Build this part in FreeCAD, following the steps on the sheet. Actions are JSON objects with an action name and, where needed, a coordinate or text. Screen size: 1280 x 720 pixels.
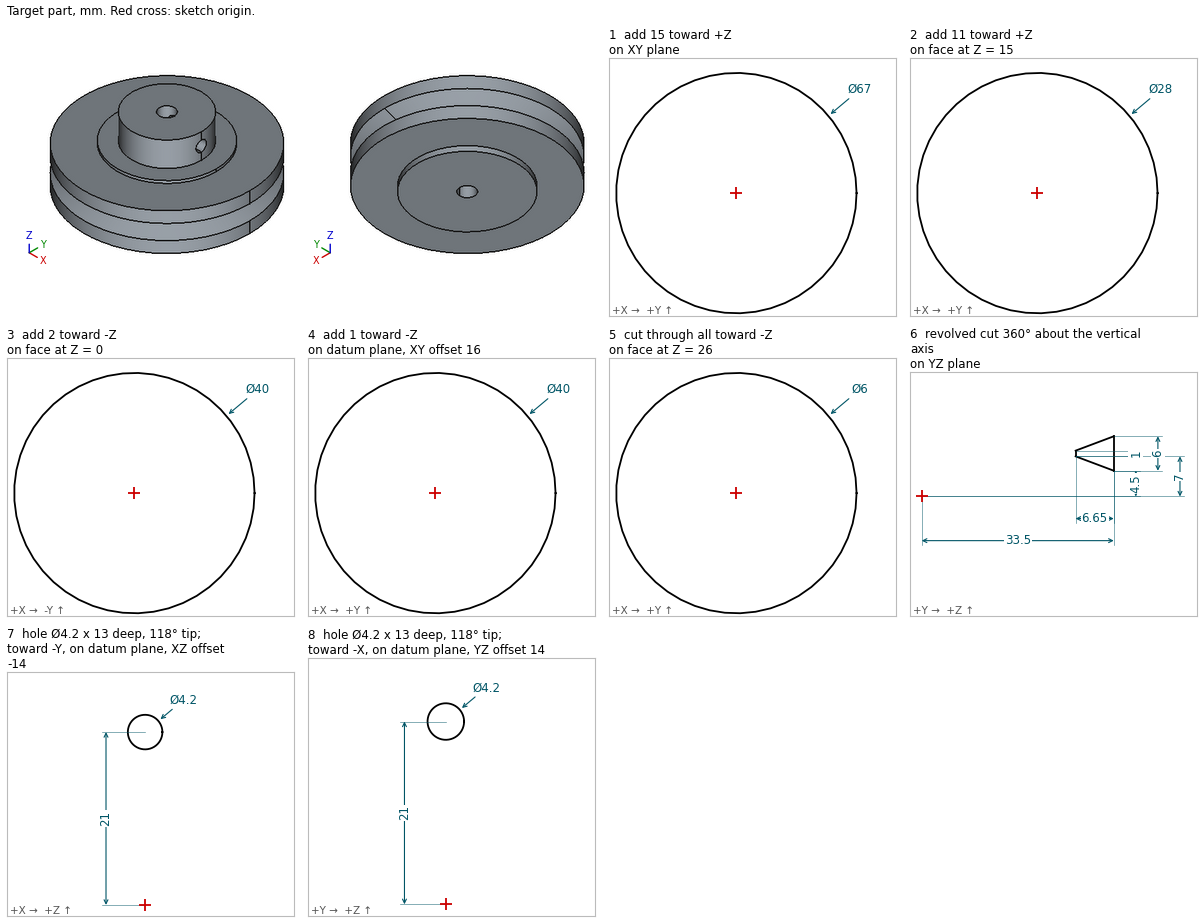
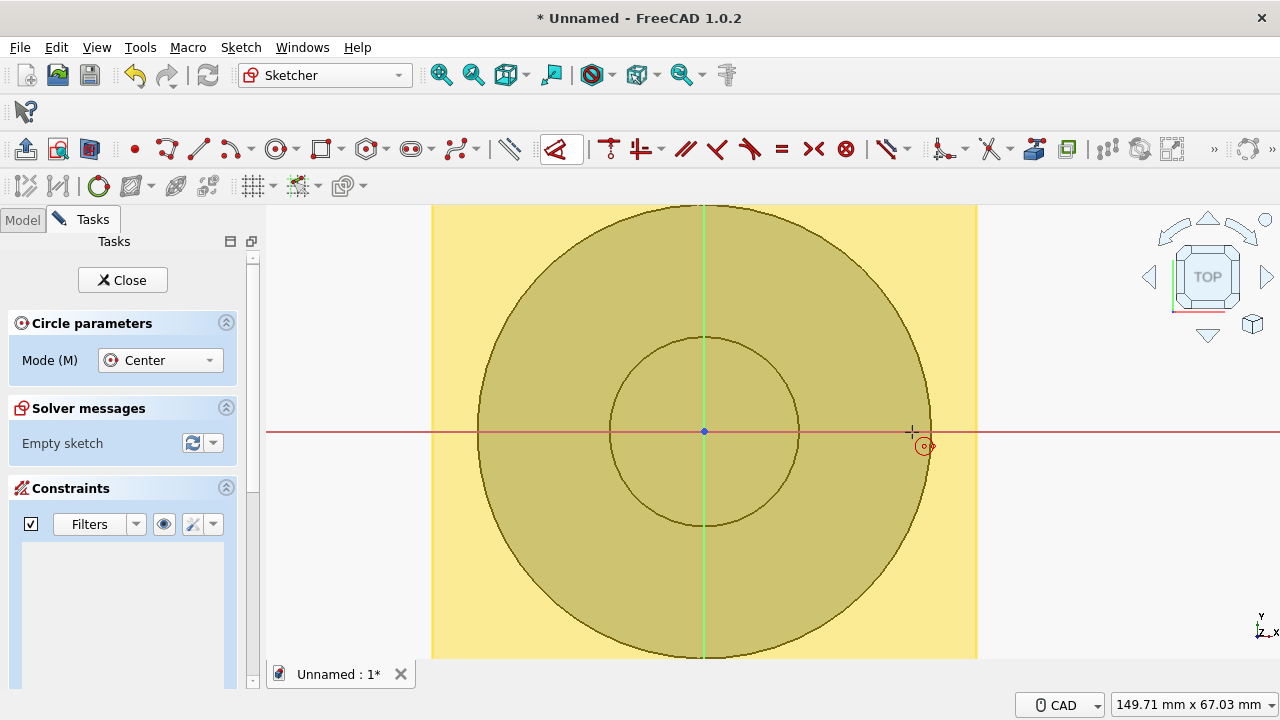
{"action": "left_click", "coordinate": [704, 432]}
{"action": "left_click", "coordinate": [800, 336]}
{"action": "key", "text": "Escape"}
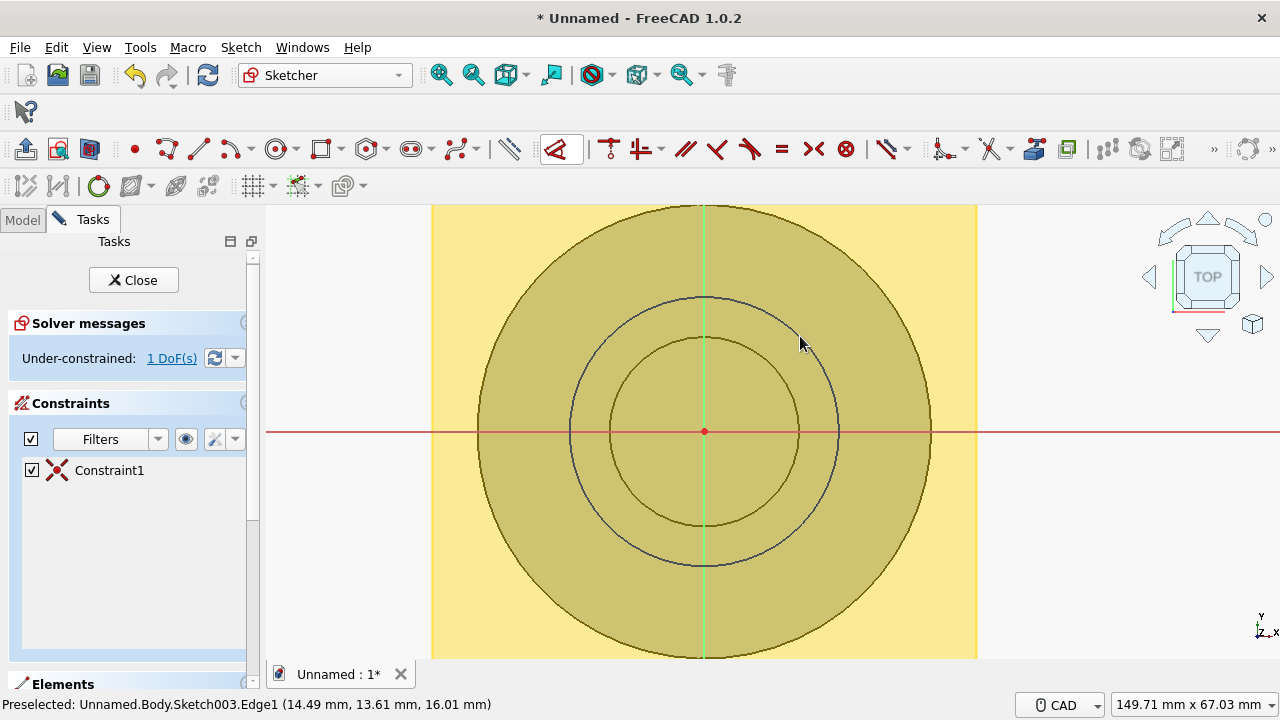
{"action": "left_click", "coordinate": [799, 336]}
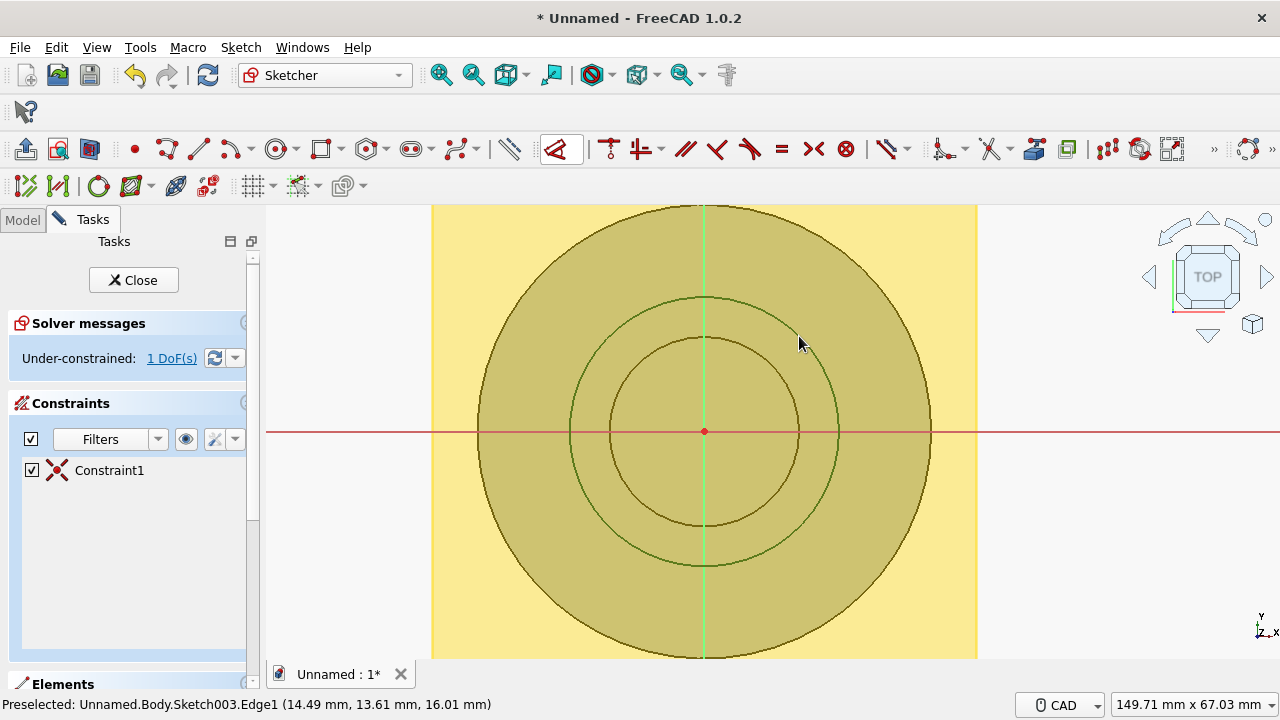
{"action": "key", "text": "k o"}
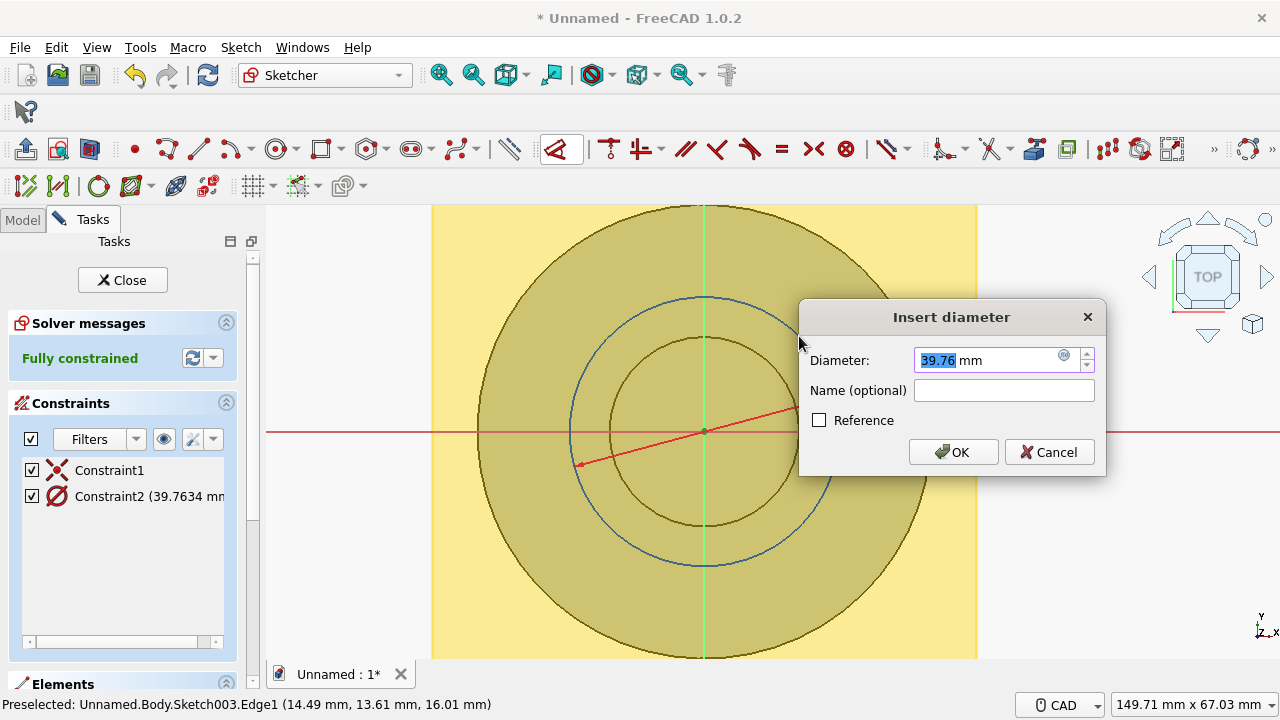
{"action": "type", "text": "40"}
{"action": "key", "text": "Return"}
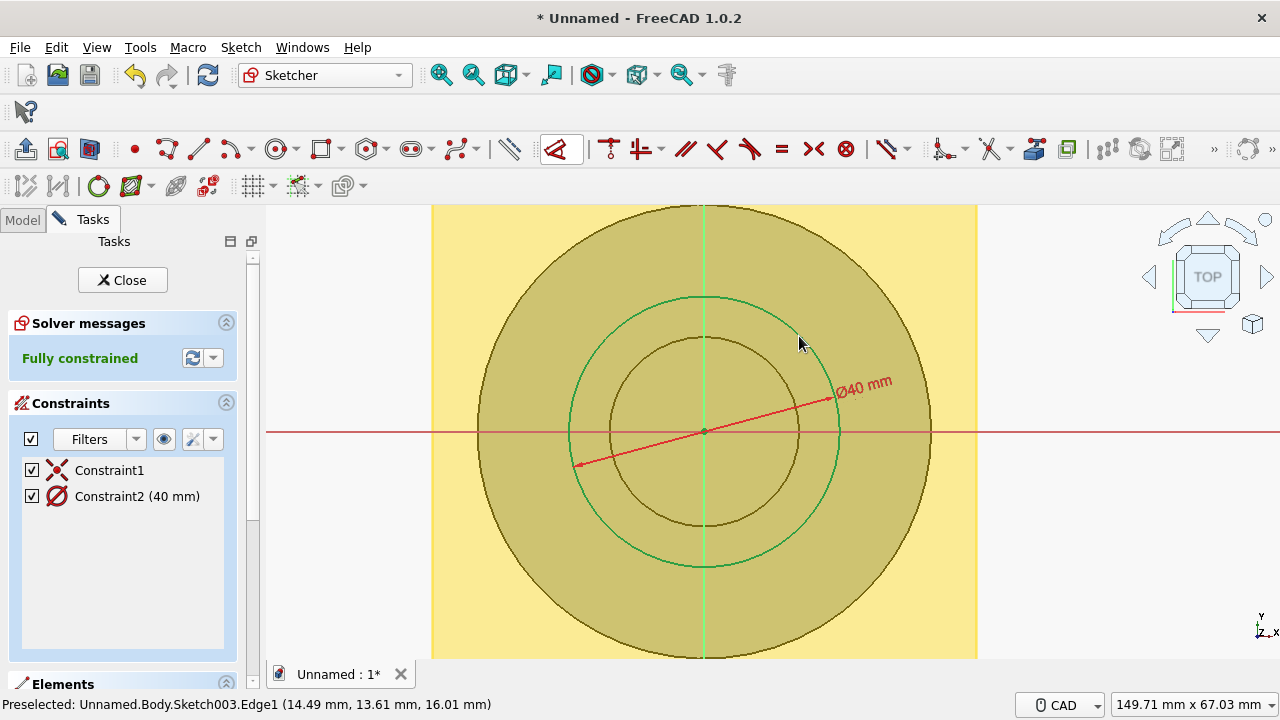
{"action": "left_click", "coordinate": [123, 280]}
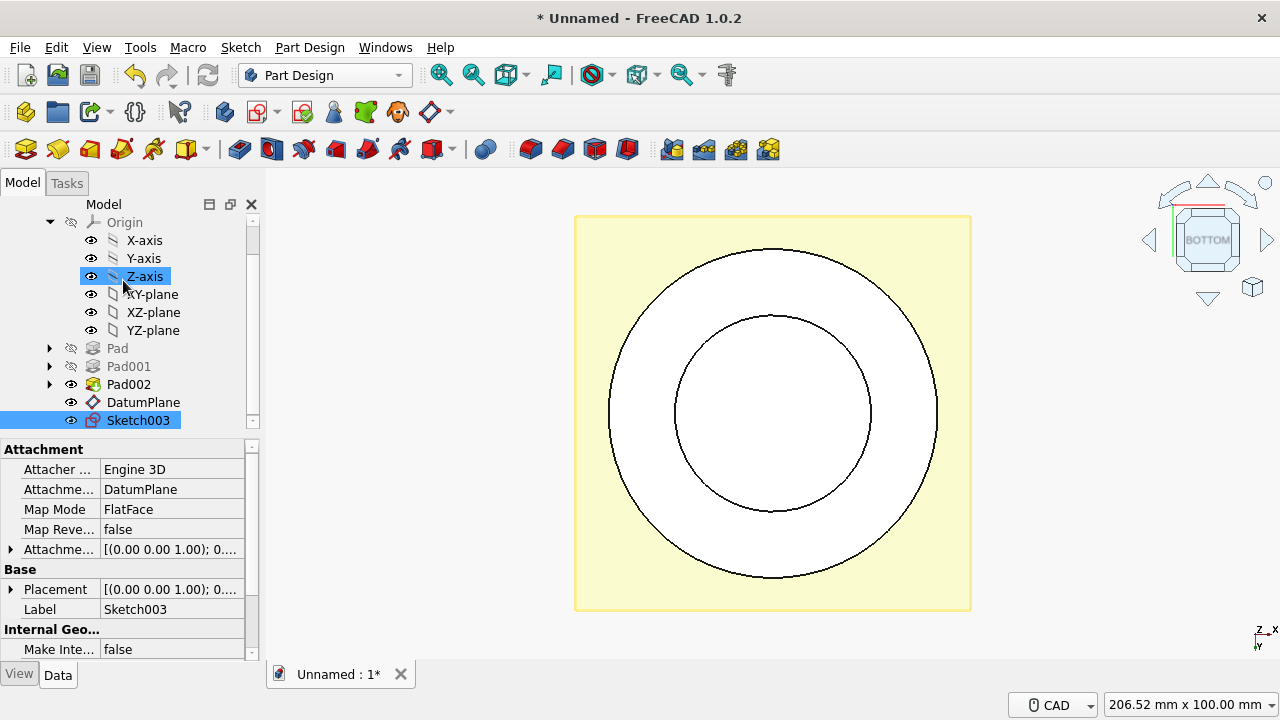
{"action": "left_click", "coordinate": [26, 150]}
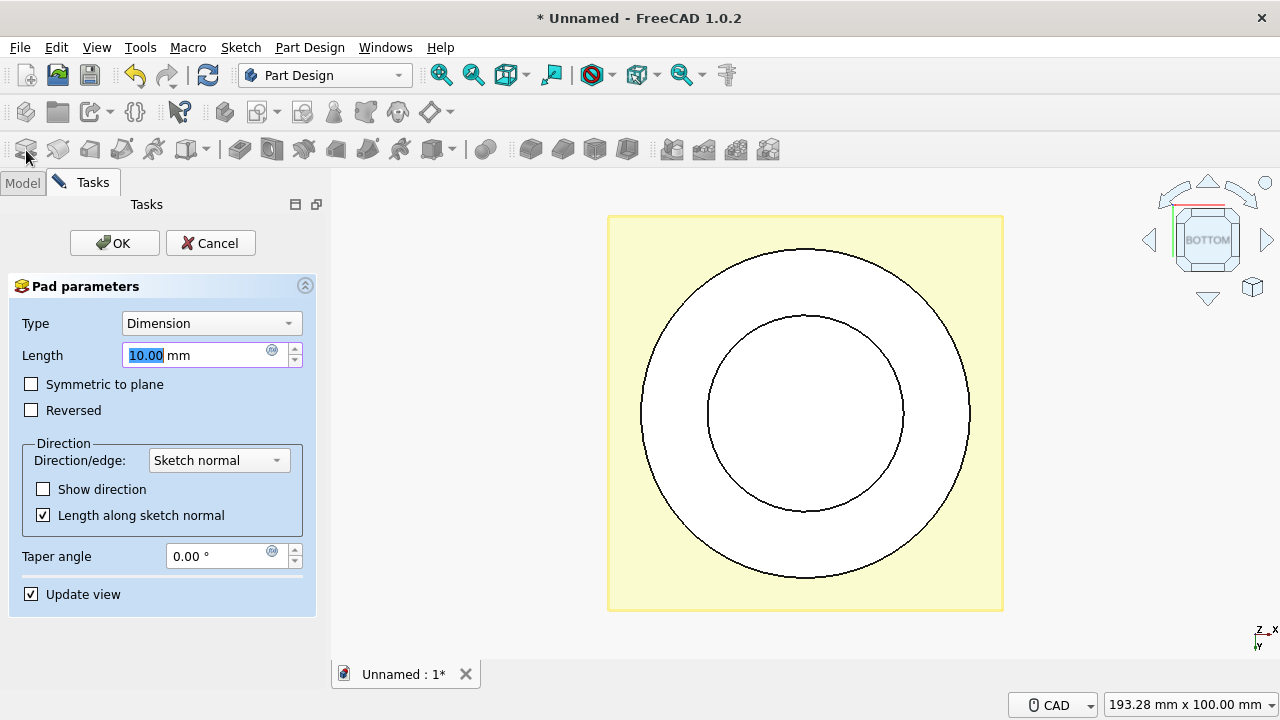
{"action": "type", "text": "1"}
{"action": "key", "text": "Tab"}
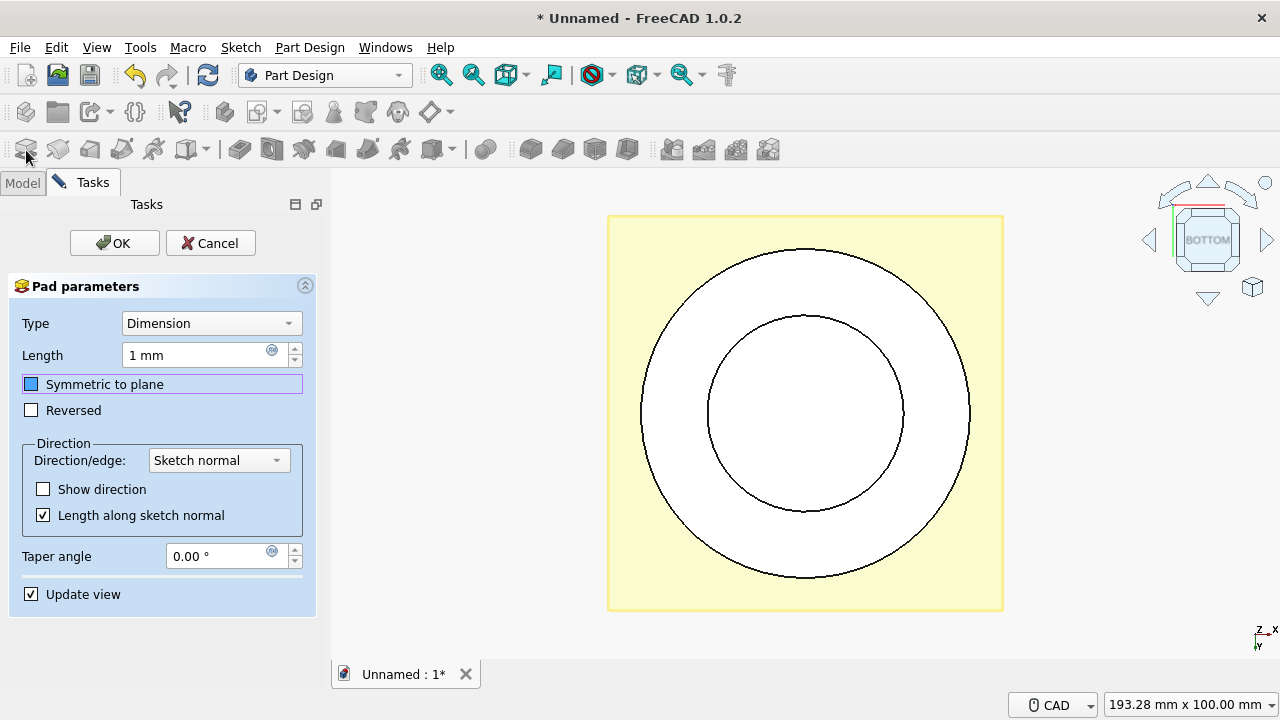
{"action": "left_click", "coordinate": [30, 410]}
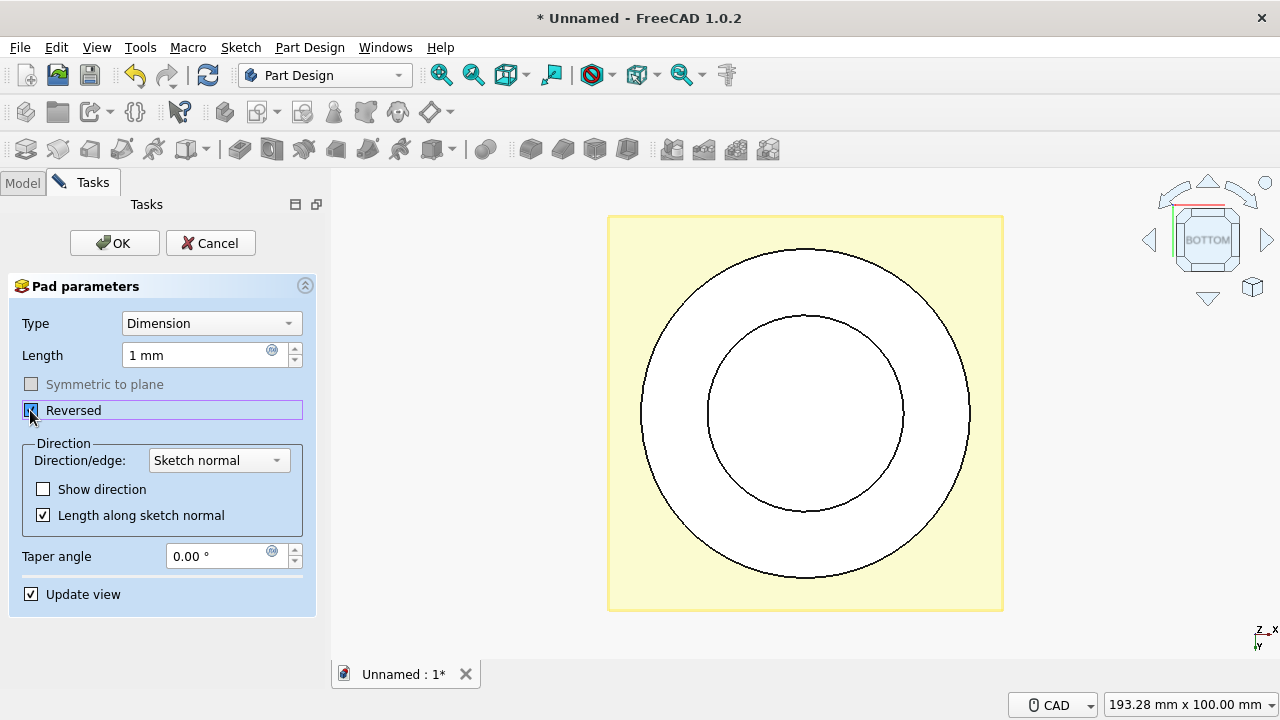
{"action": "left_click", "coordinate": [115, 243]}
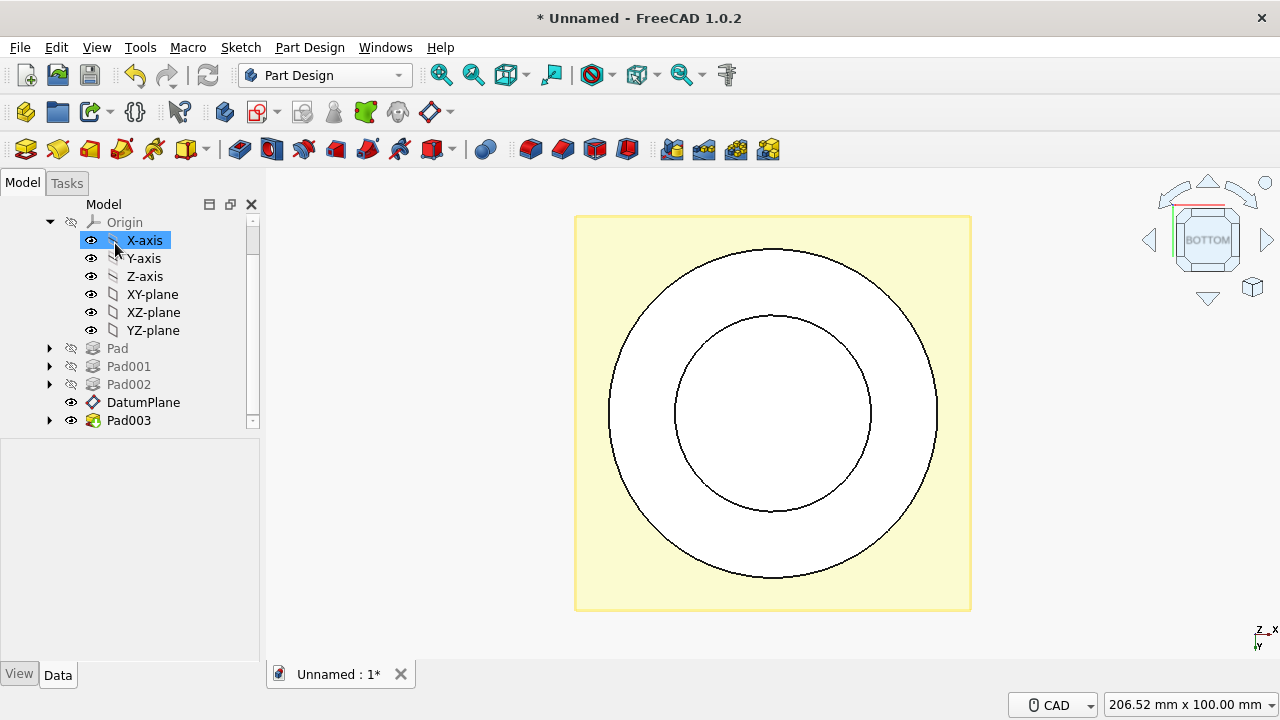
{"action": "left_click", "coordinate": [116, 402]}
{"action": "key", "text": "space"}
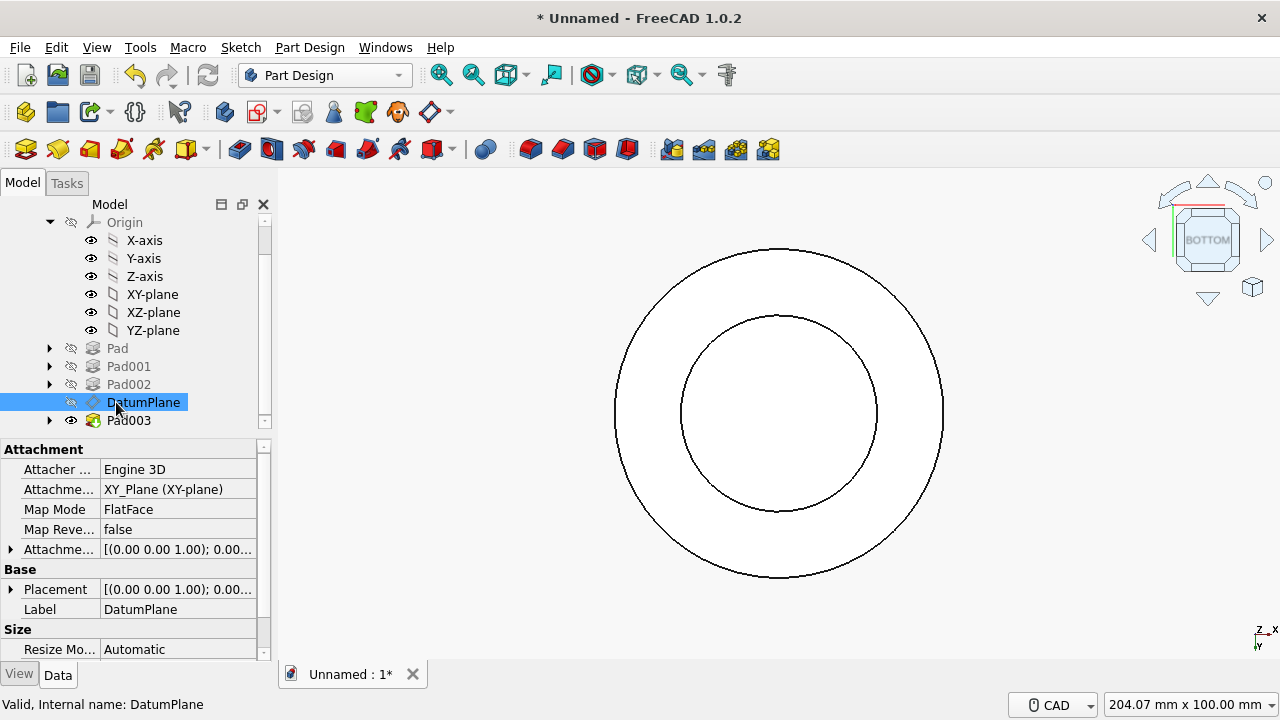
{"action": "key", "text": "0"}